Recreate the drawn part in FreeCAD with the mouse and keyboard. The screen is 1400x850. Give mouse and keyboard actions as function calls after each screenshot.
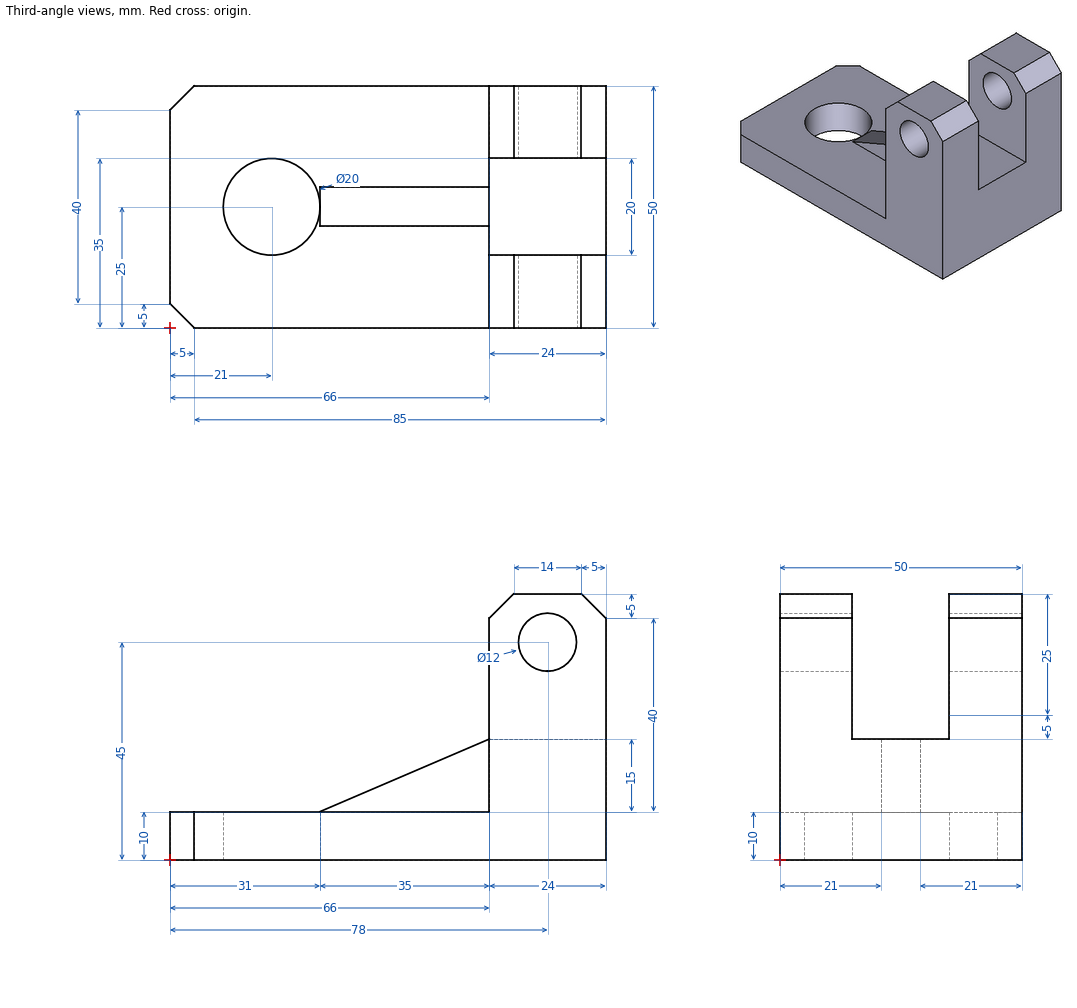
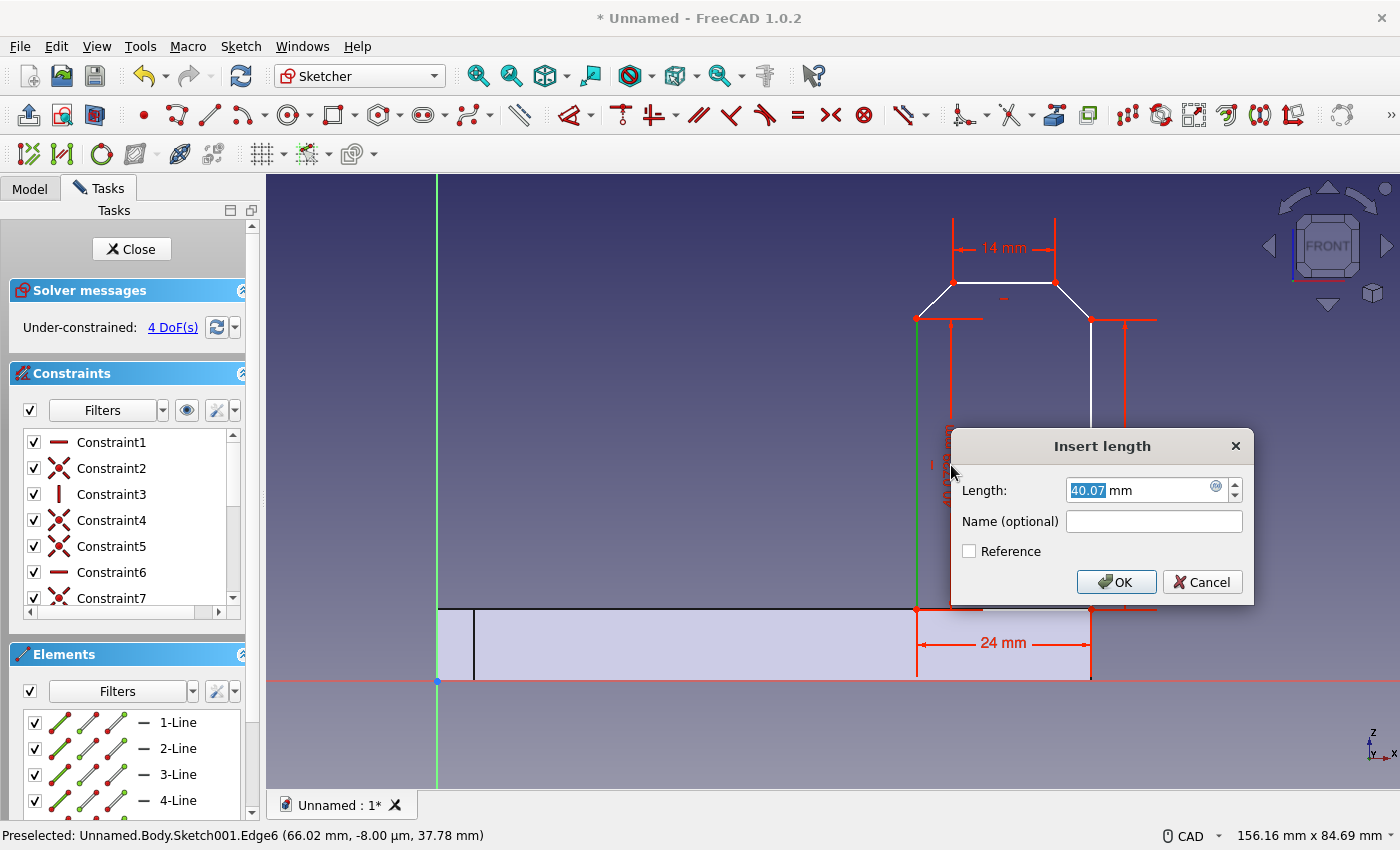
text(40)
key(Return)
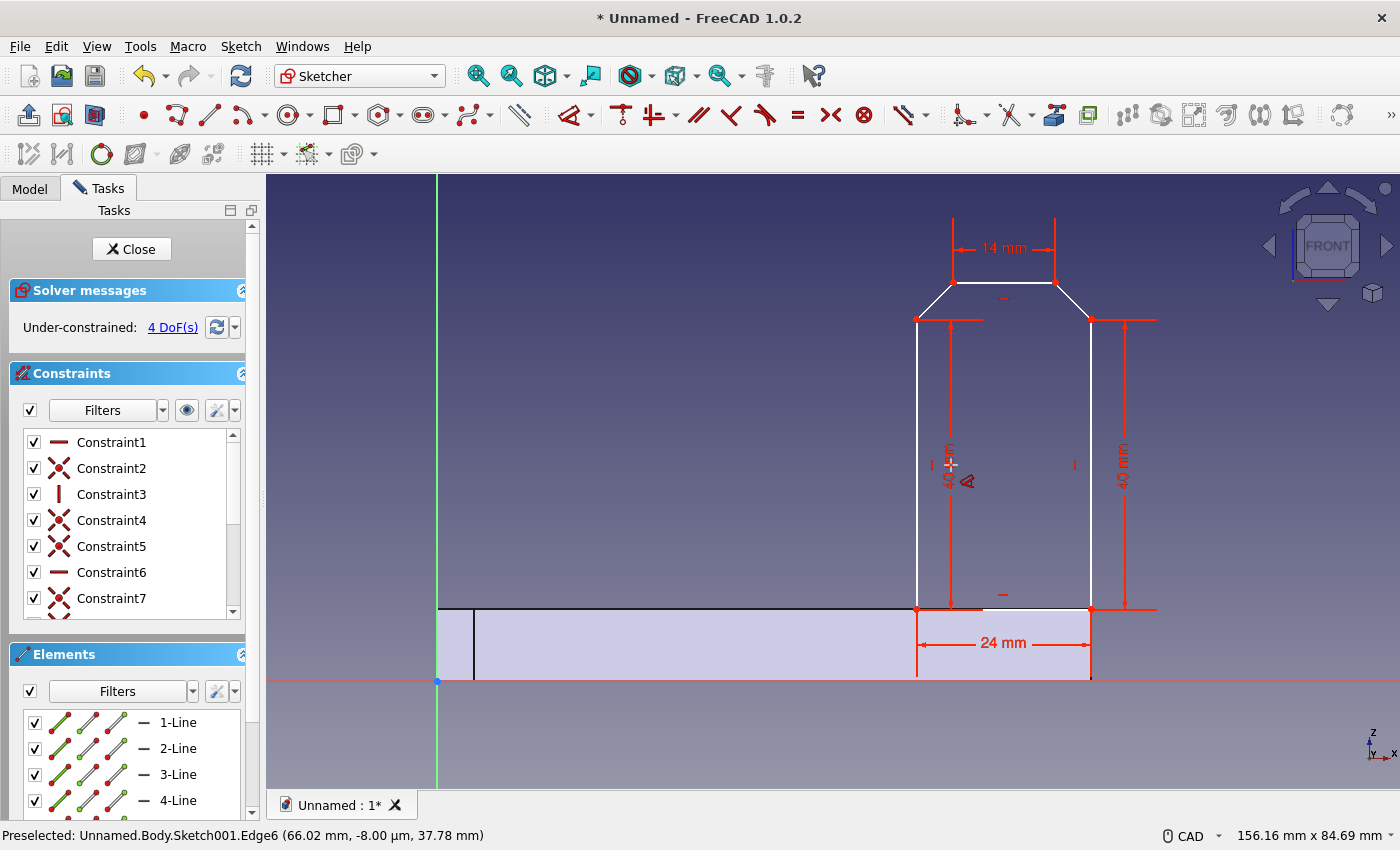
click(1080, 309)
click(1081, 249)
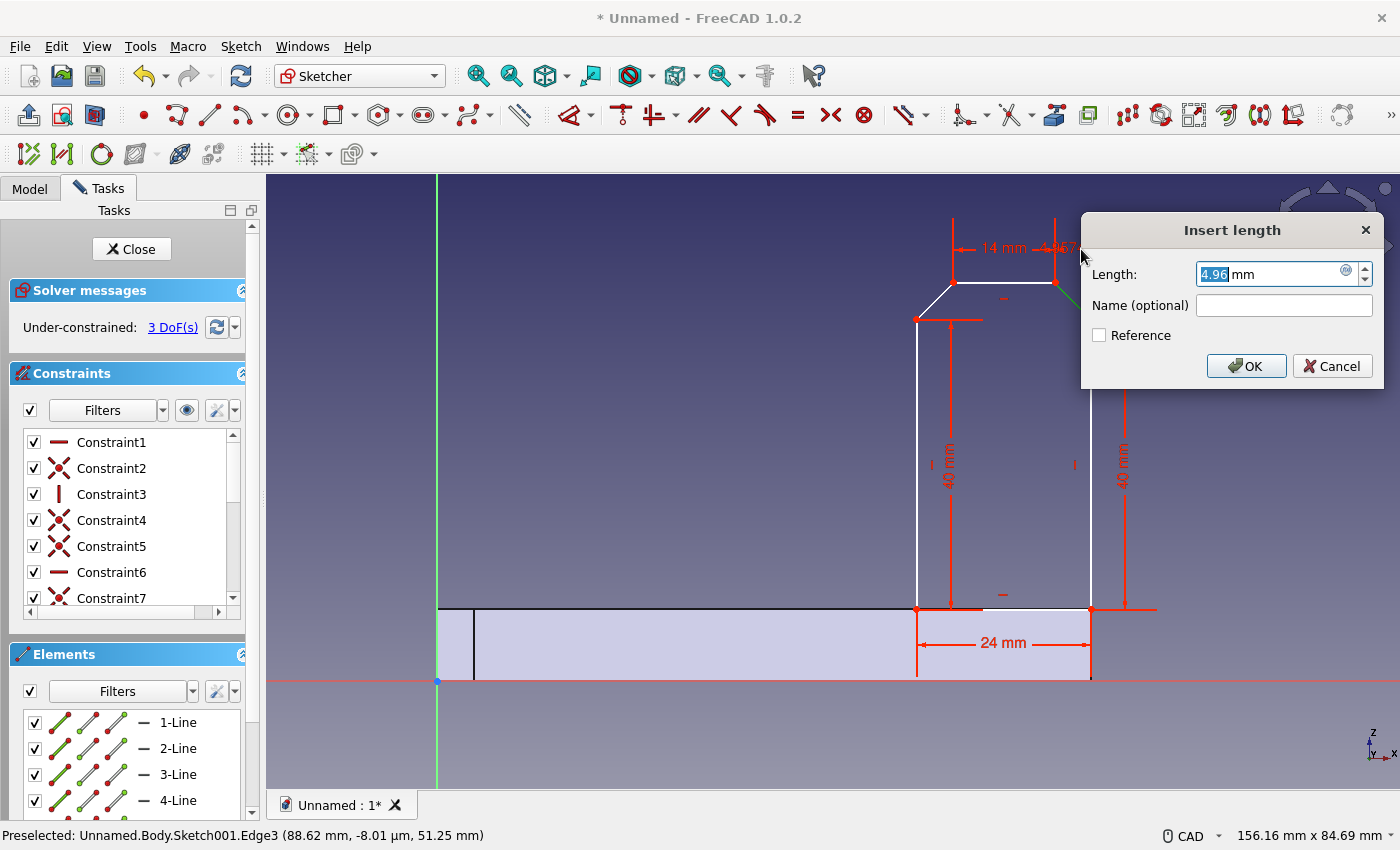
text(5)
key(Return)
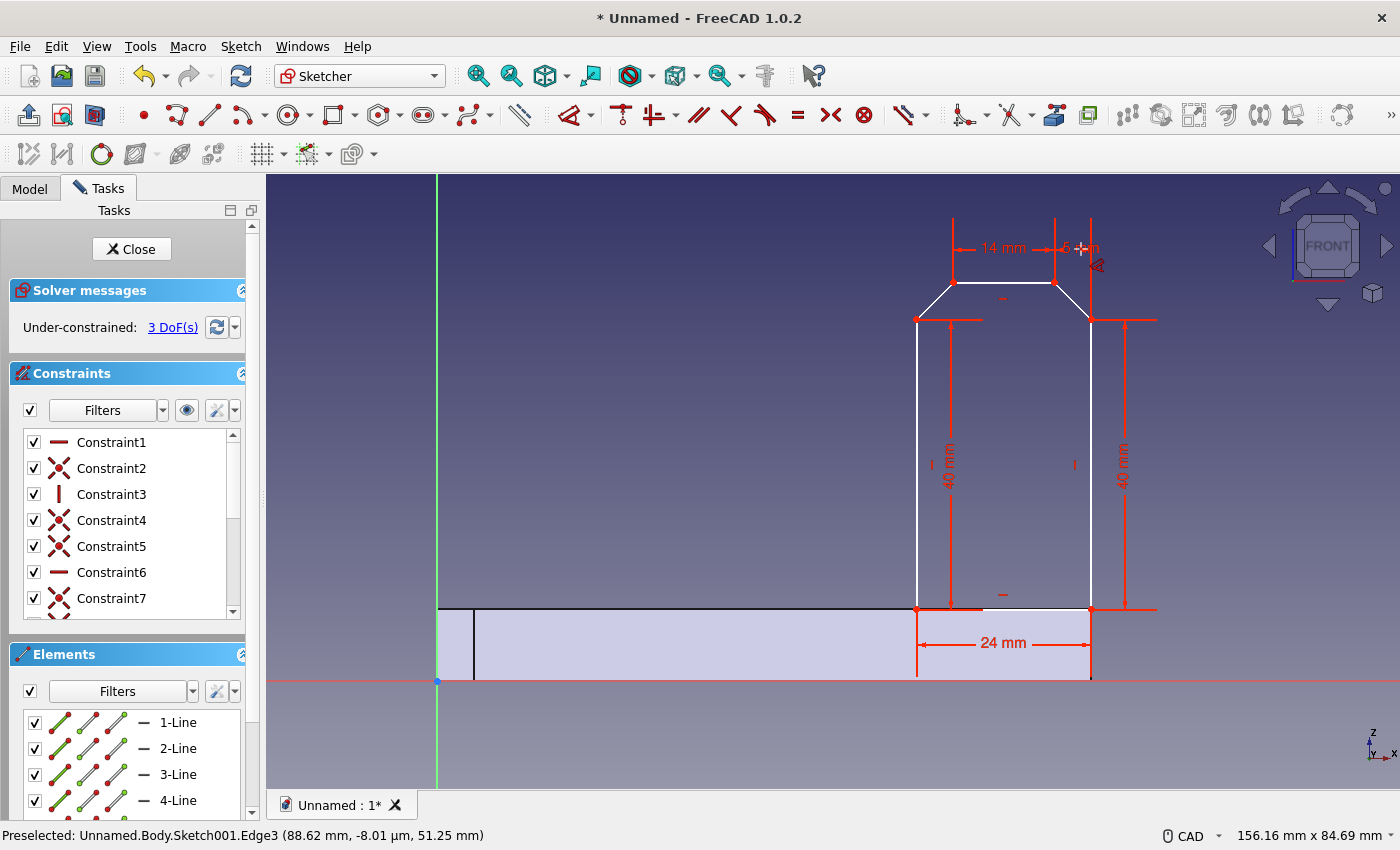
click(1080, 309)
click(1125, 301)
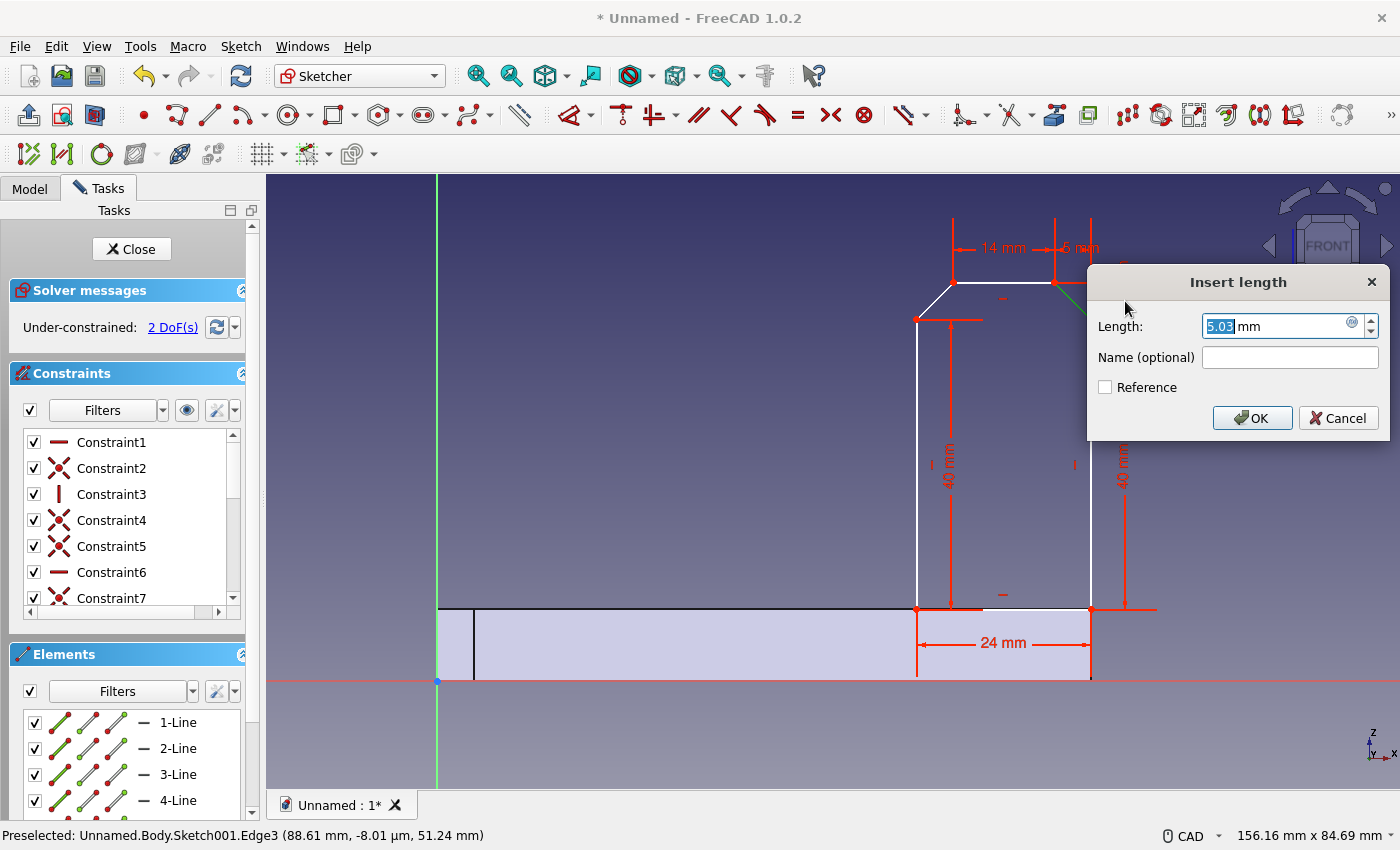
text(5)
key(Return)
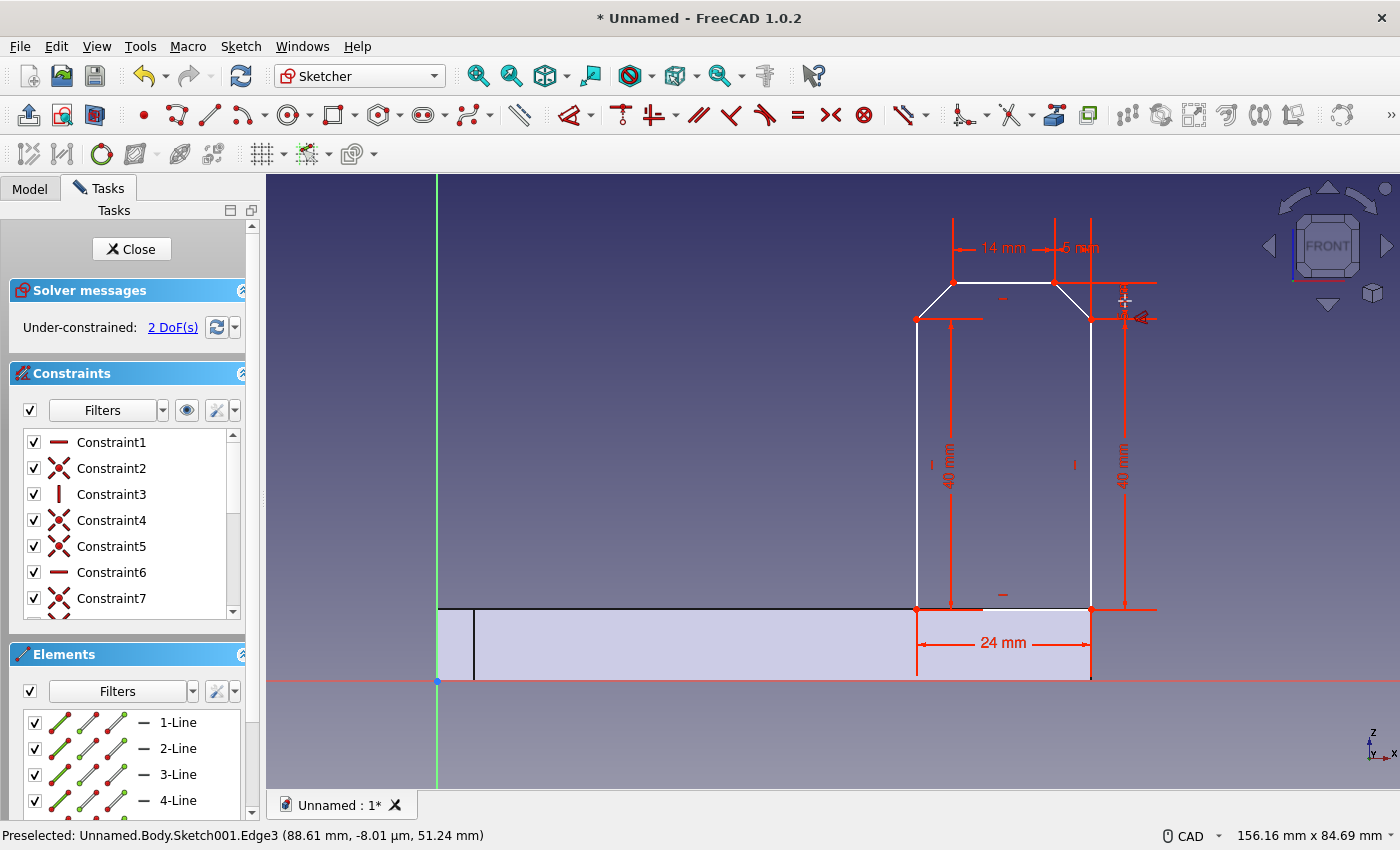
click(917, 610)
click(677, 715)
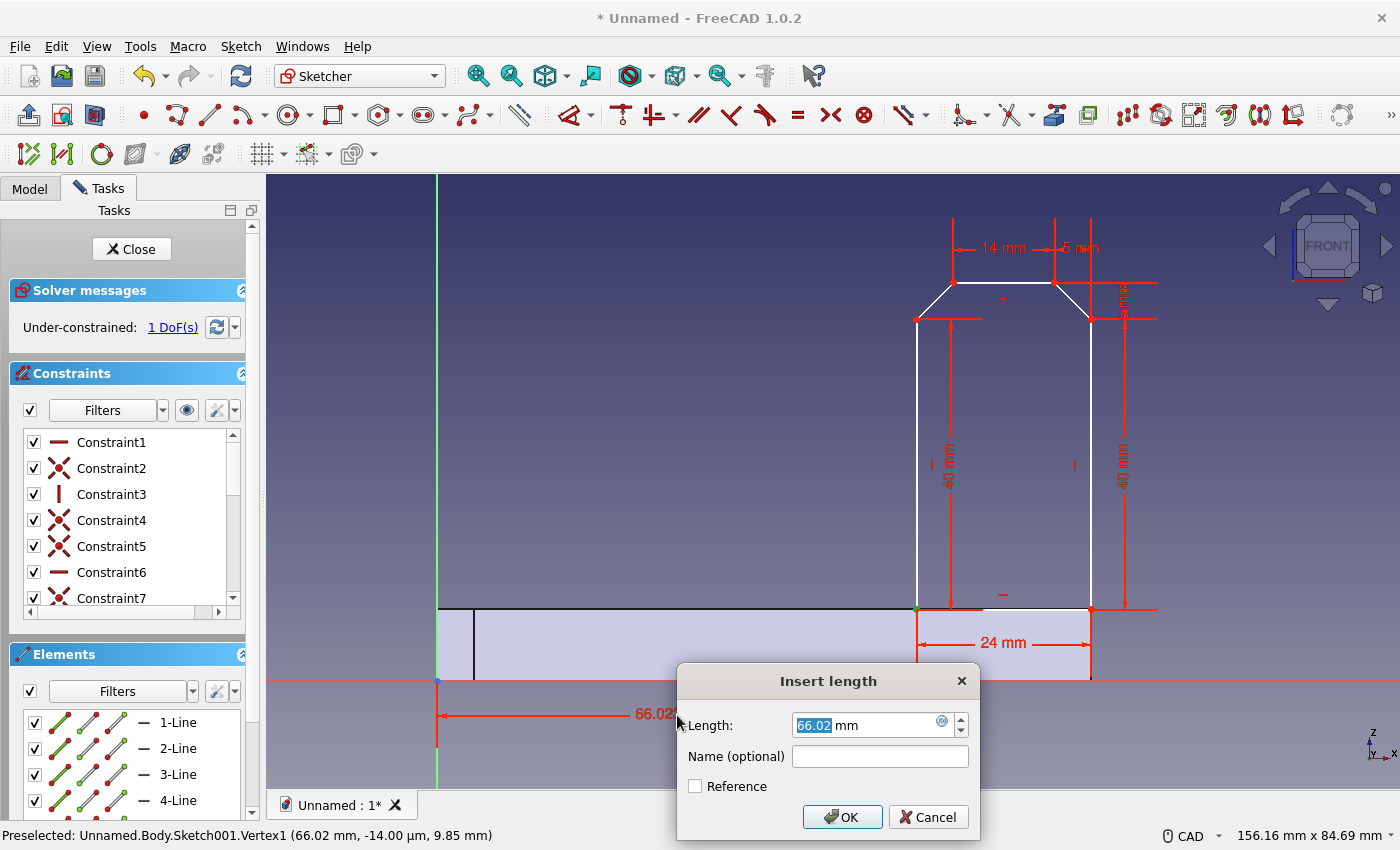
text(66)
key(Return)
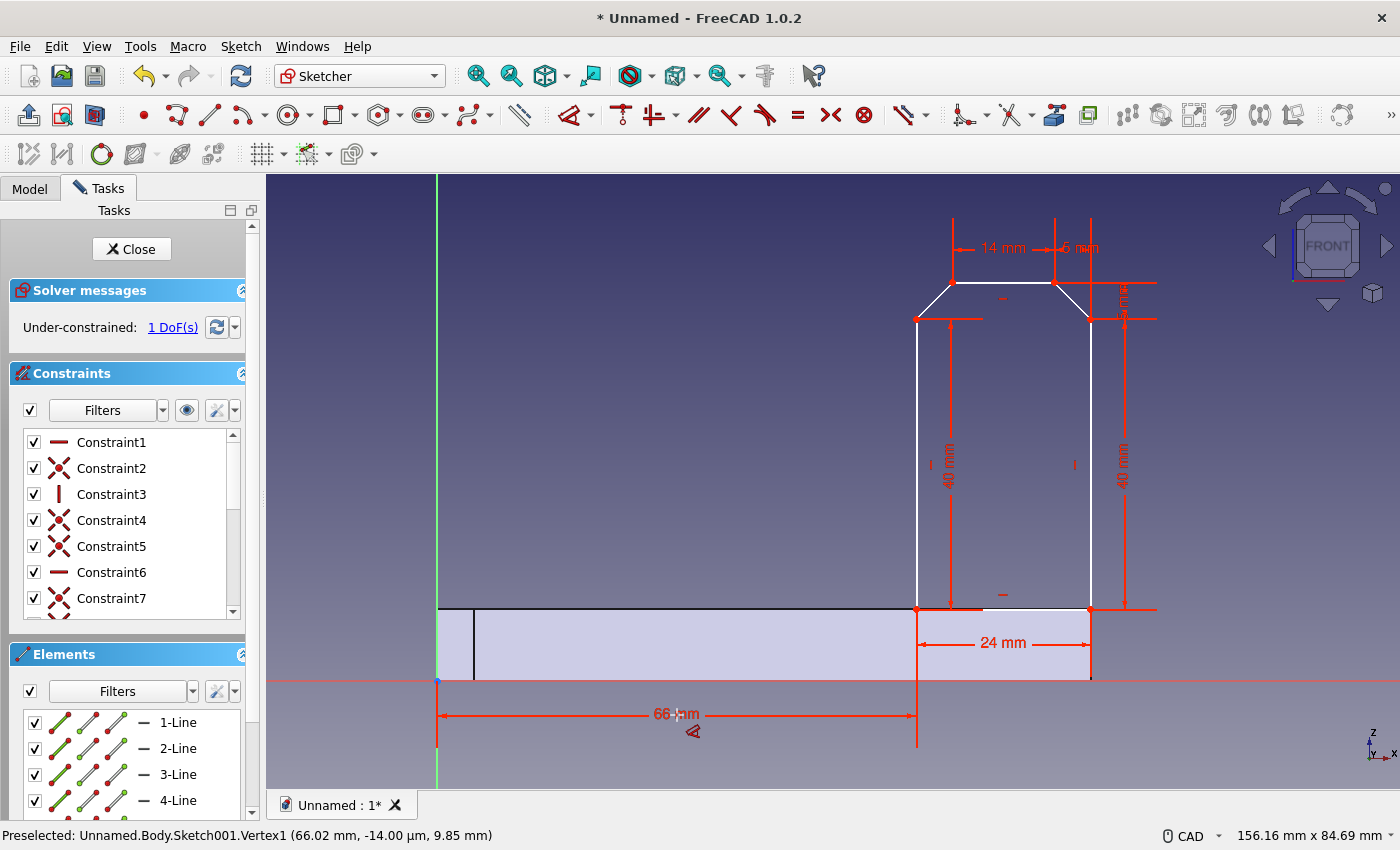
click(917, 610)
click(403, 646)